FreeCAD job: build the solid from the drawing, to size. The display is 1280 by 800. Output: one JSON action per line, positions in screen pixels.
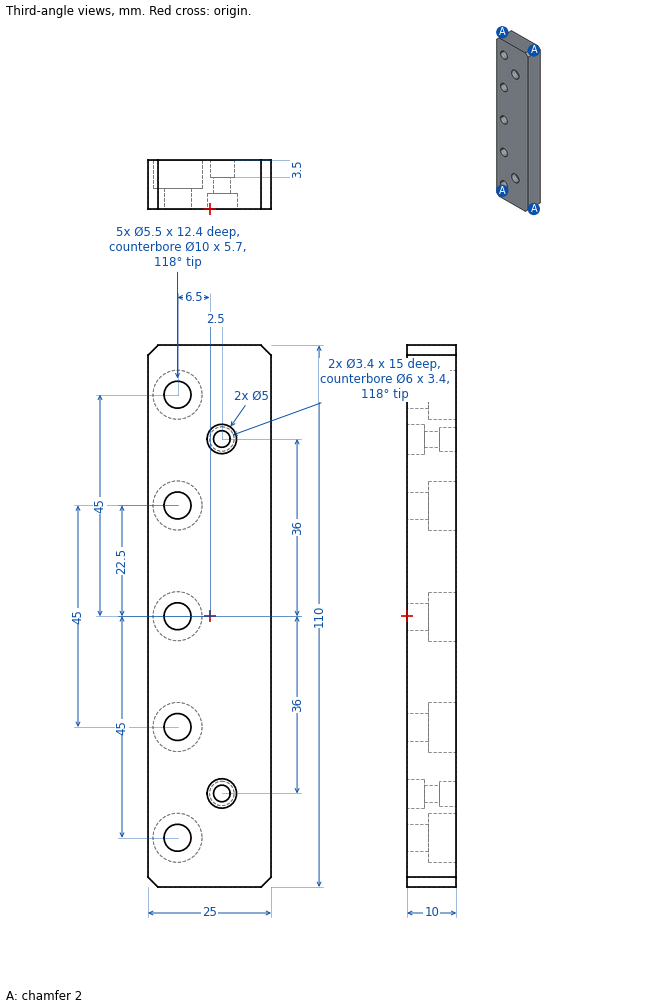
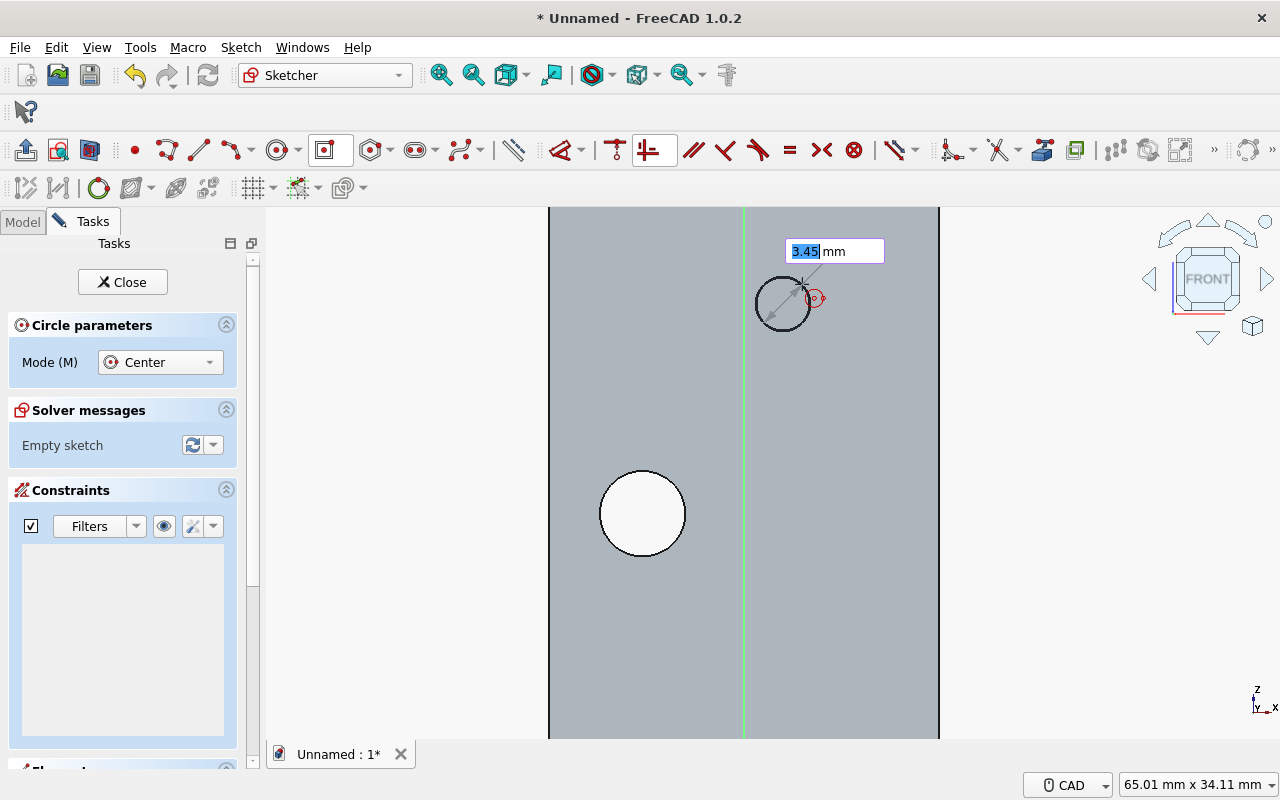
{"action": "type", "text": "3.4"}
{"action": "key", "text": "Return"}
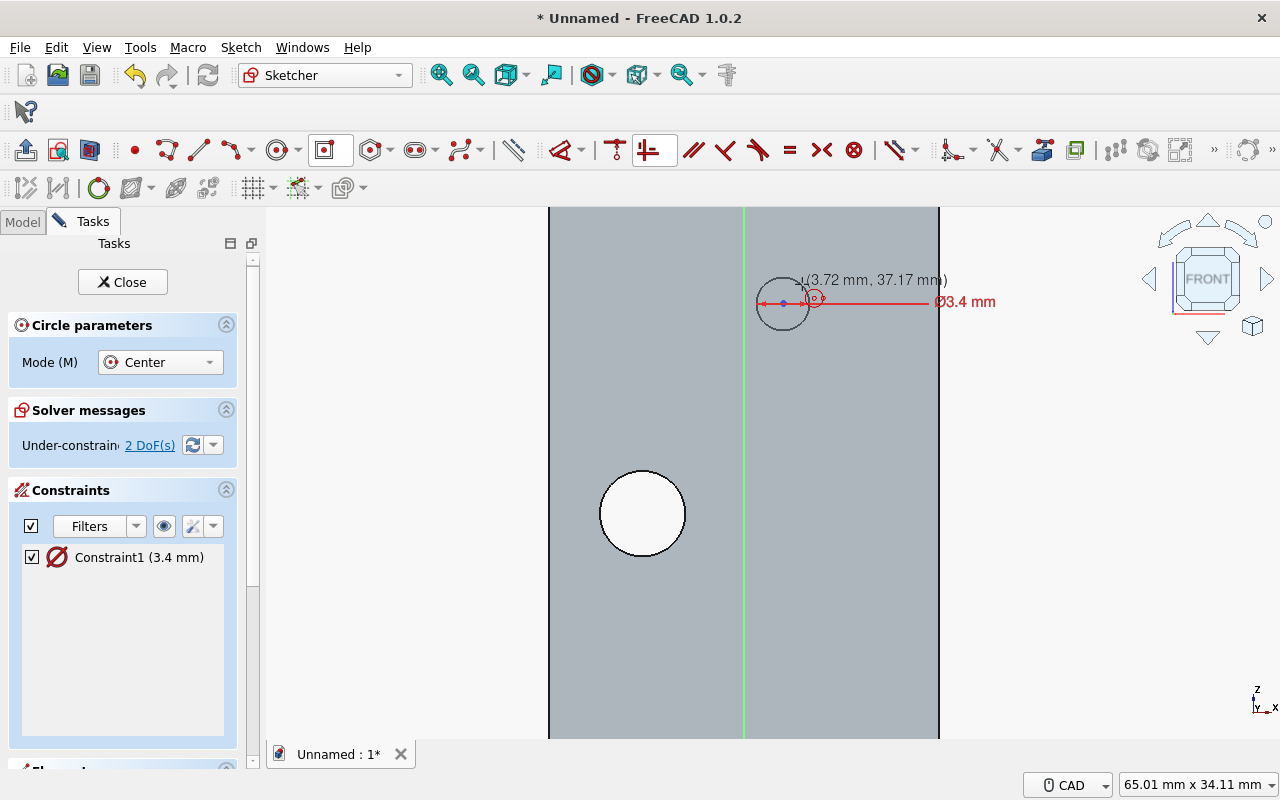
{"action": "scroll", "coordinate": [673, 304], "scroll_direction": "down", "scroll_amount": 6}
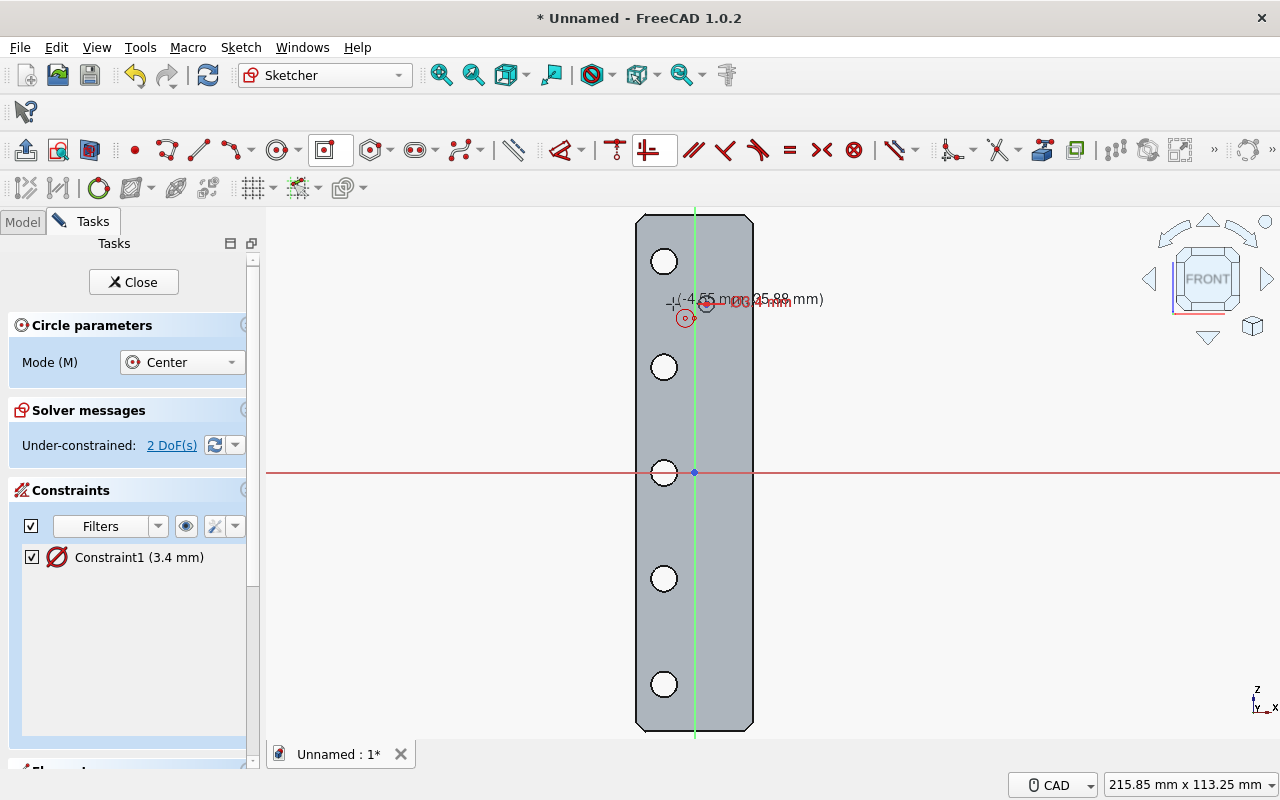
{"action": "scroll", "coordinate": [706, 642], "scroll_direction": "up", "scroll_amount": 6}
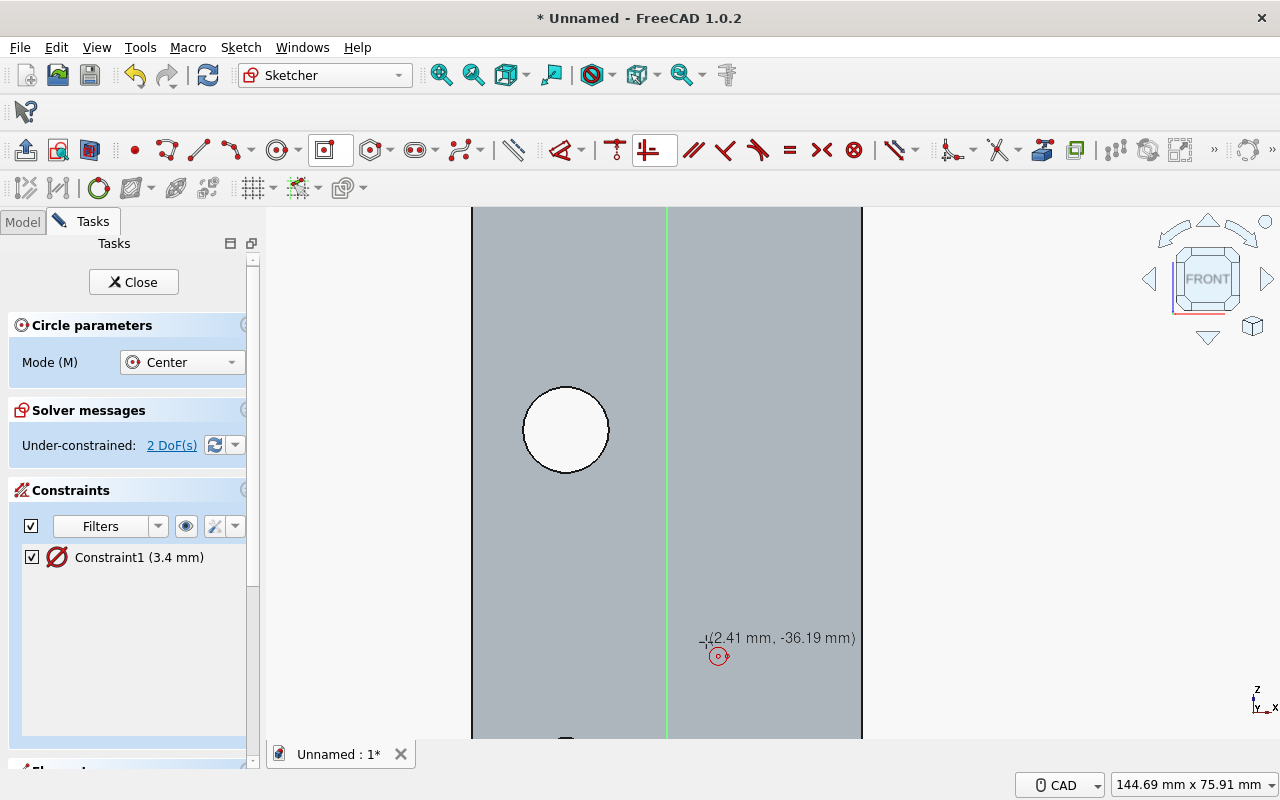
{"action": "left_click", "coordinate": [706, 640]}
{"action": "mouse_move", "coordinate": [725, 622]}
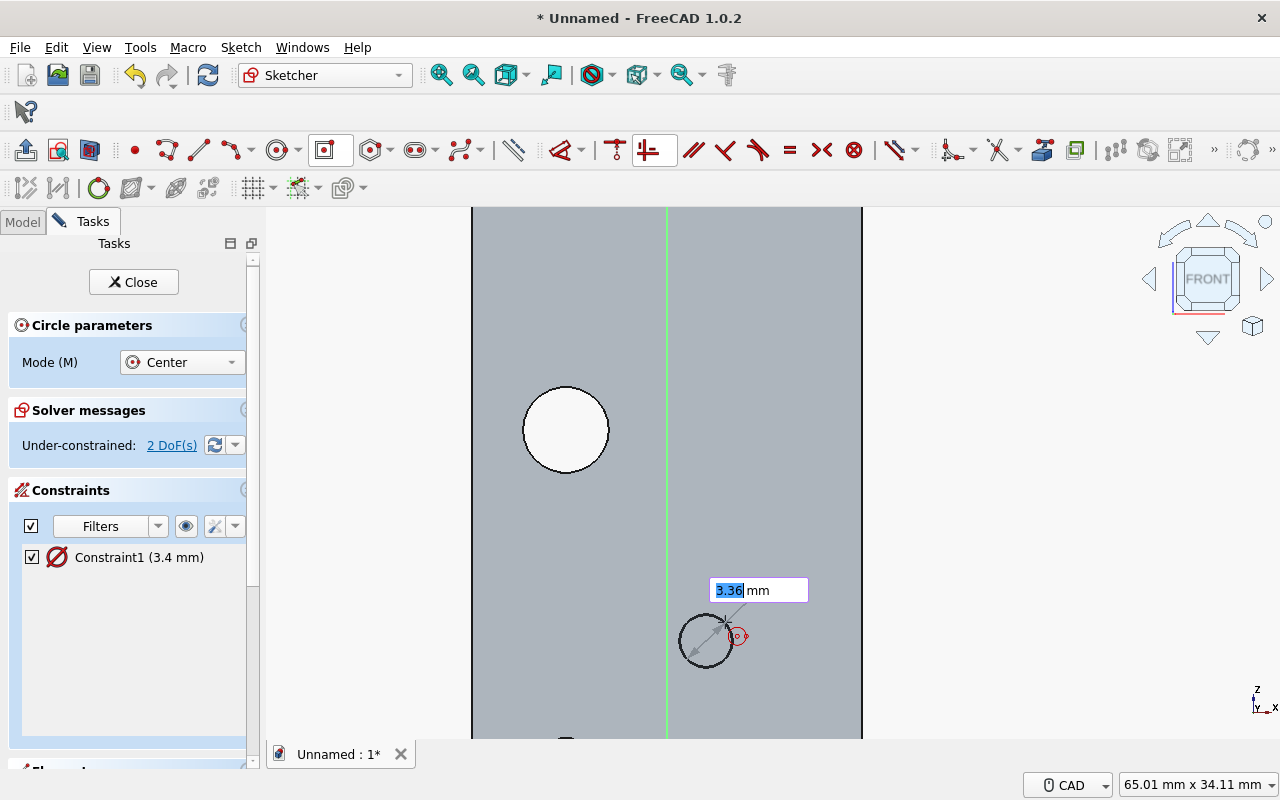
{"action": "type", "text": "3.4"}
{"action": "key", "text": "Return"}
{"action": "key", "text": "Escape"}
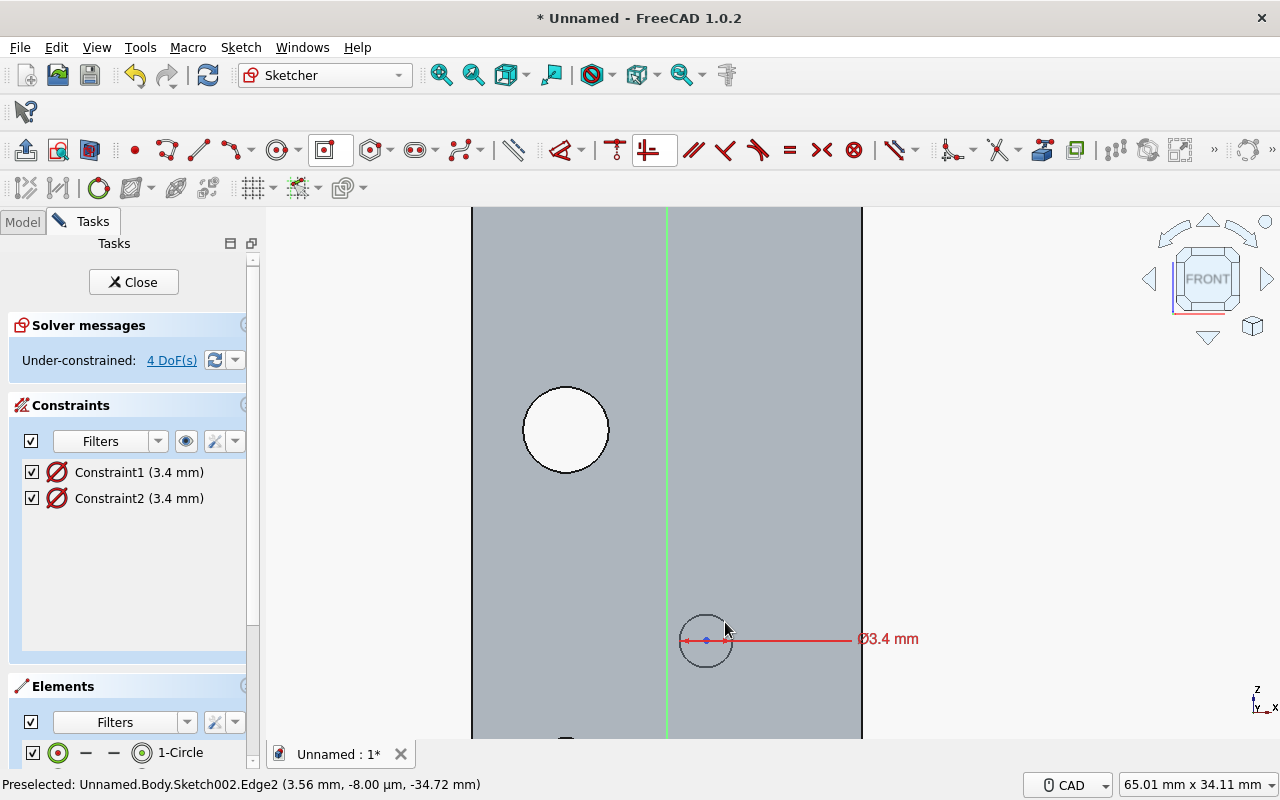
{"action": "scroll", "coordinate": [706, 643], "scroll_direction": "down", "scroll_amount": 6}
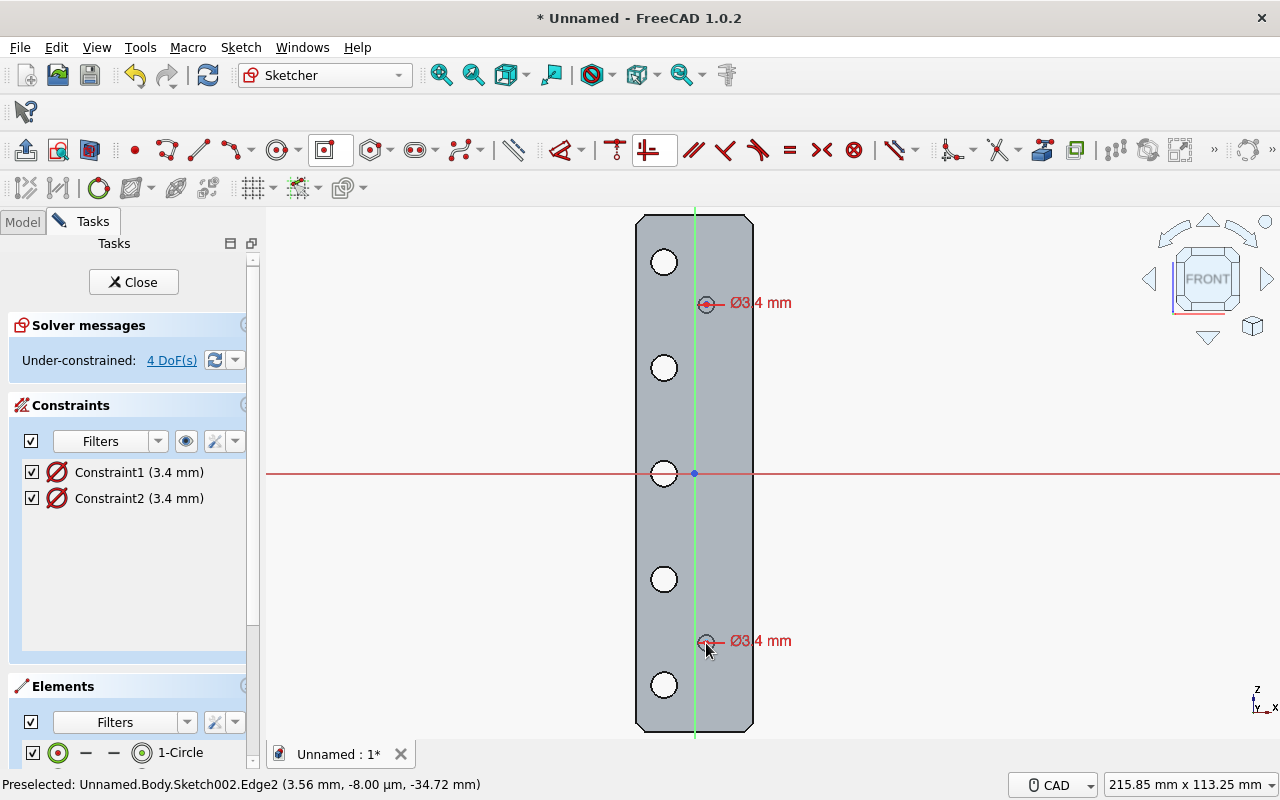
{"action": "left_click", "coordinate": [706, 305]}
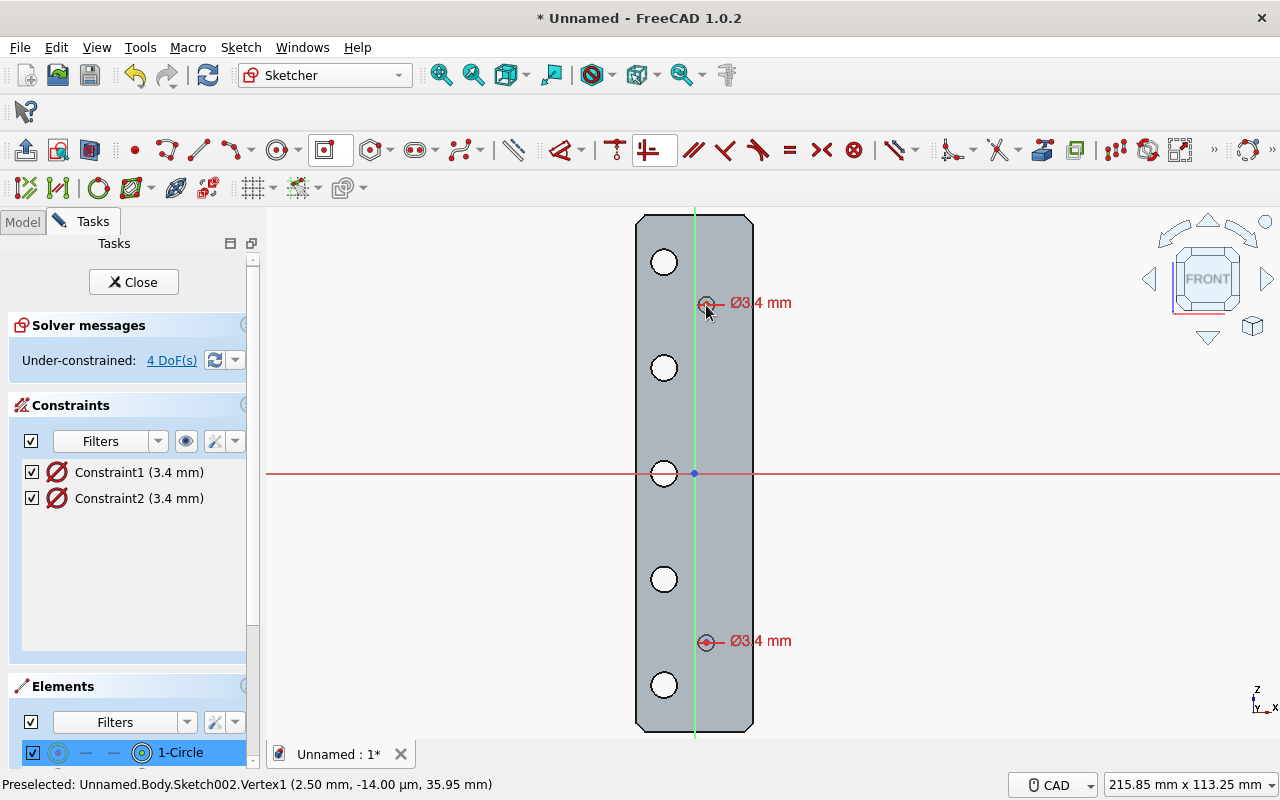
{"action": "left_click", "coordinate": [706, 643]}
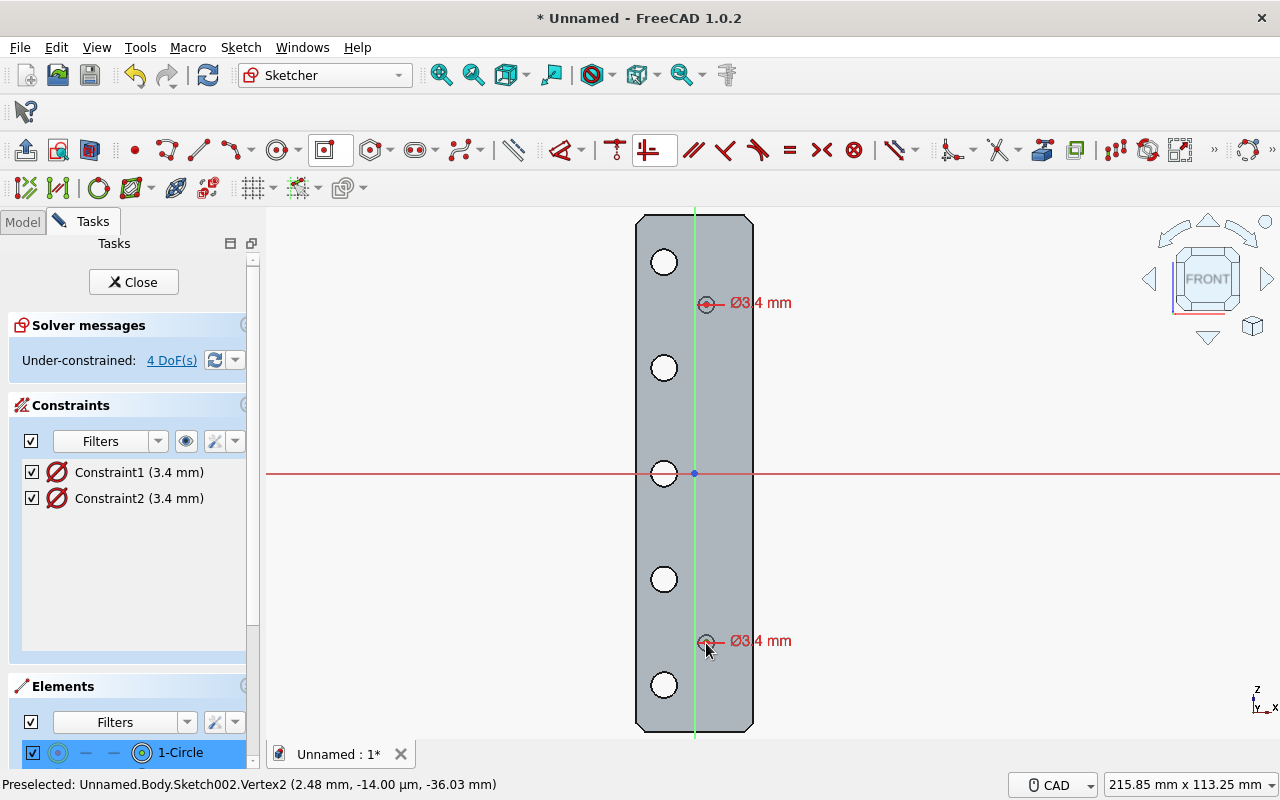
{"action": "key", "text": "v"}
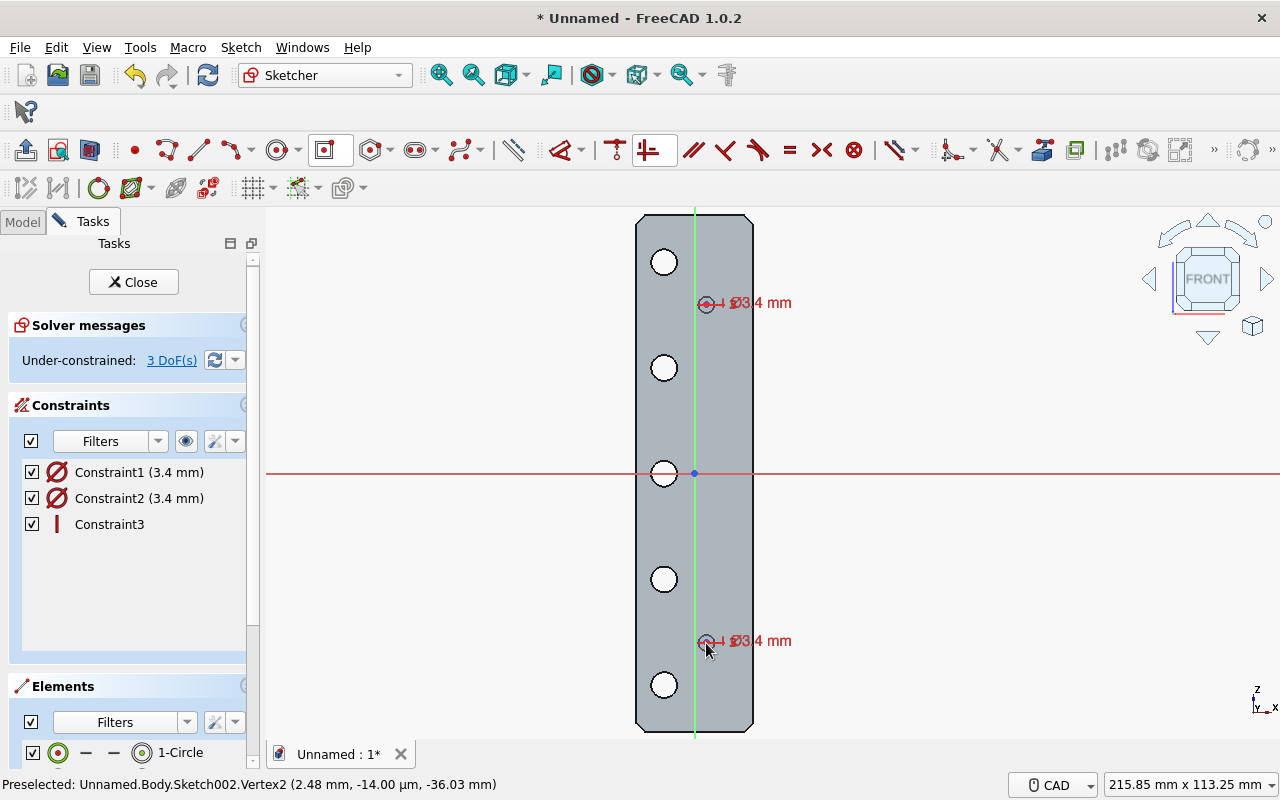
{"action": "left_click", "coordinate": [560, 150]}